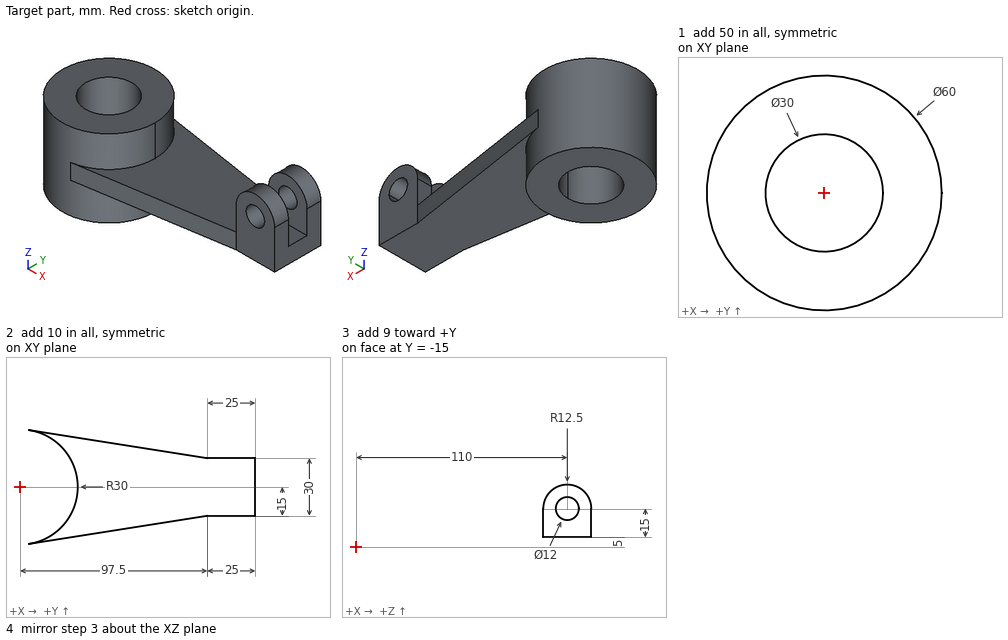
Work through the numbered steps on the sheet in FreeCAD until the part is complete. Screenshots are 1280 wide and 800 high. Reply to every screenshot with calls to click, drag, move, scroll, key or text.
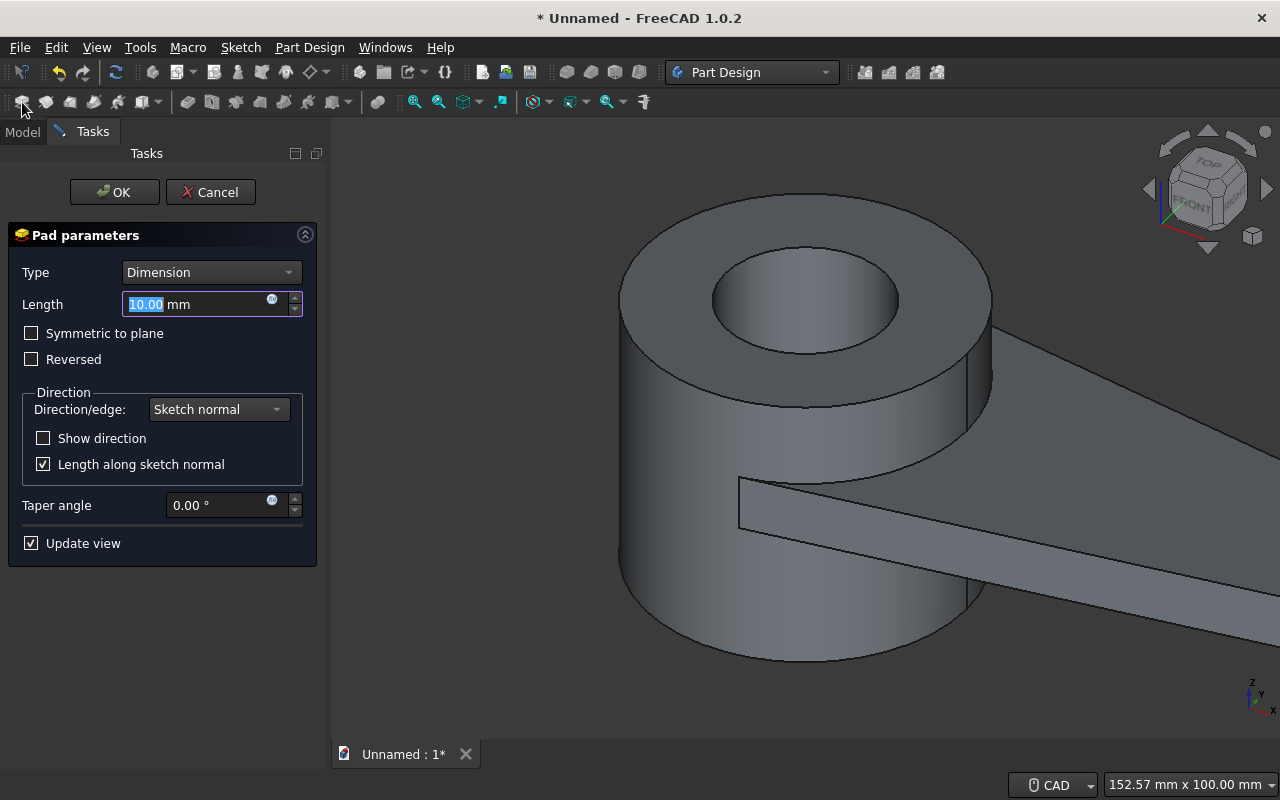
text(10)
key(Tab)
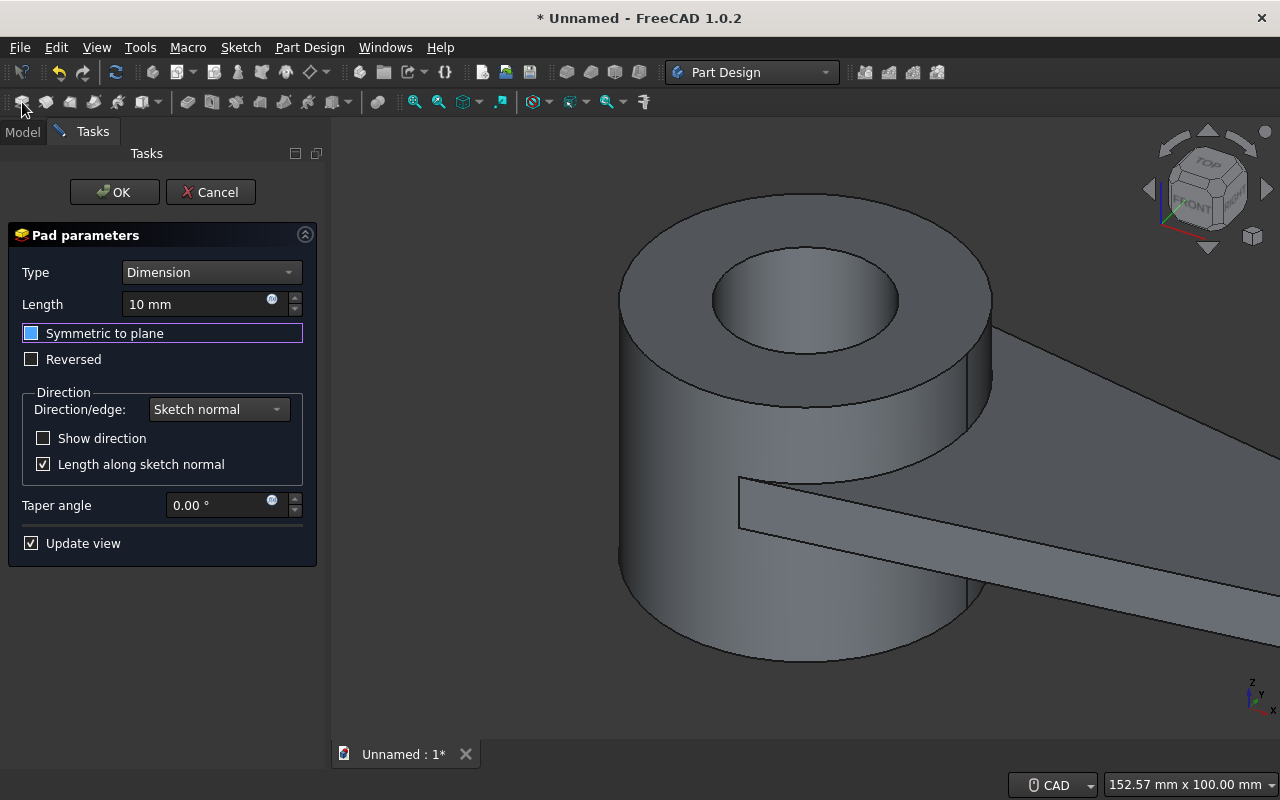
click(30, 333)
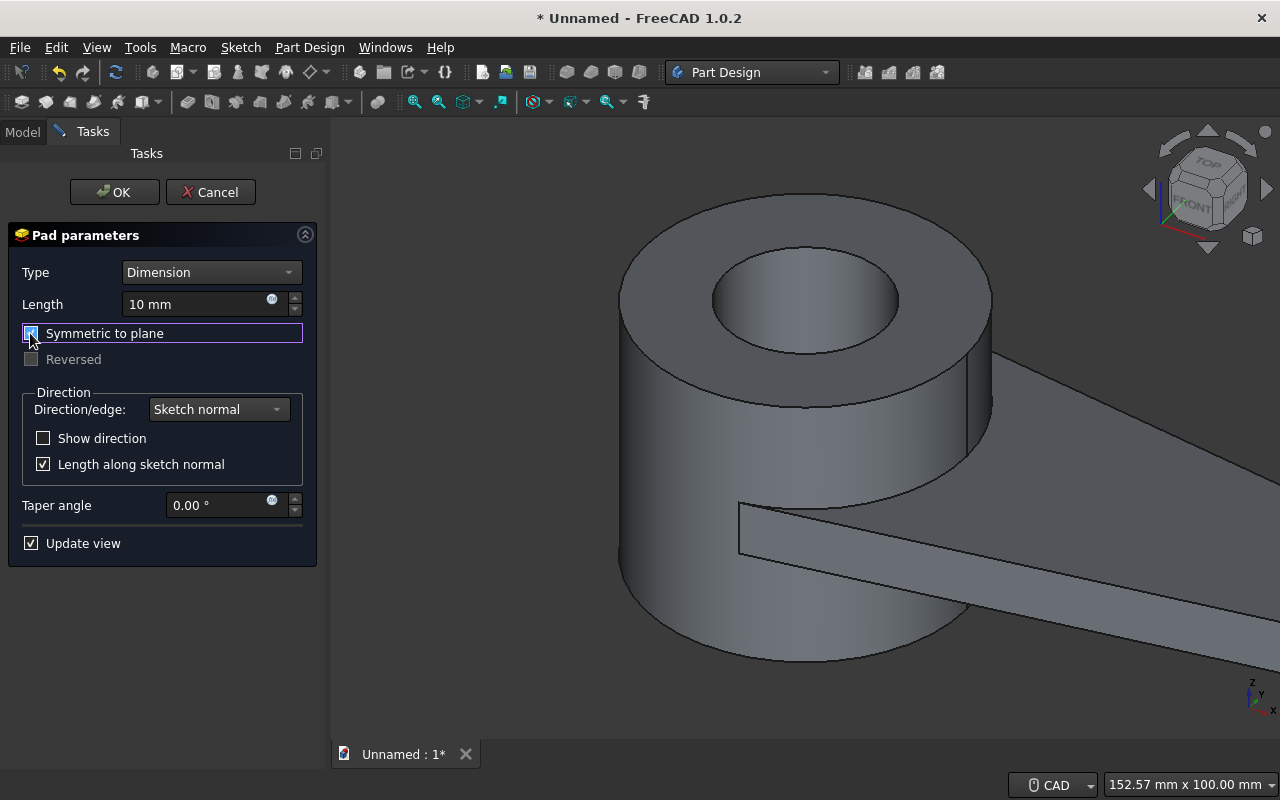
click(115, 192)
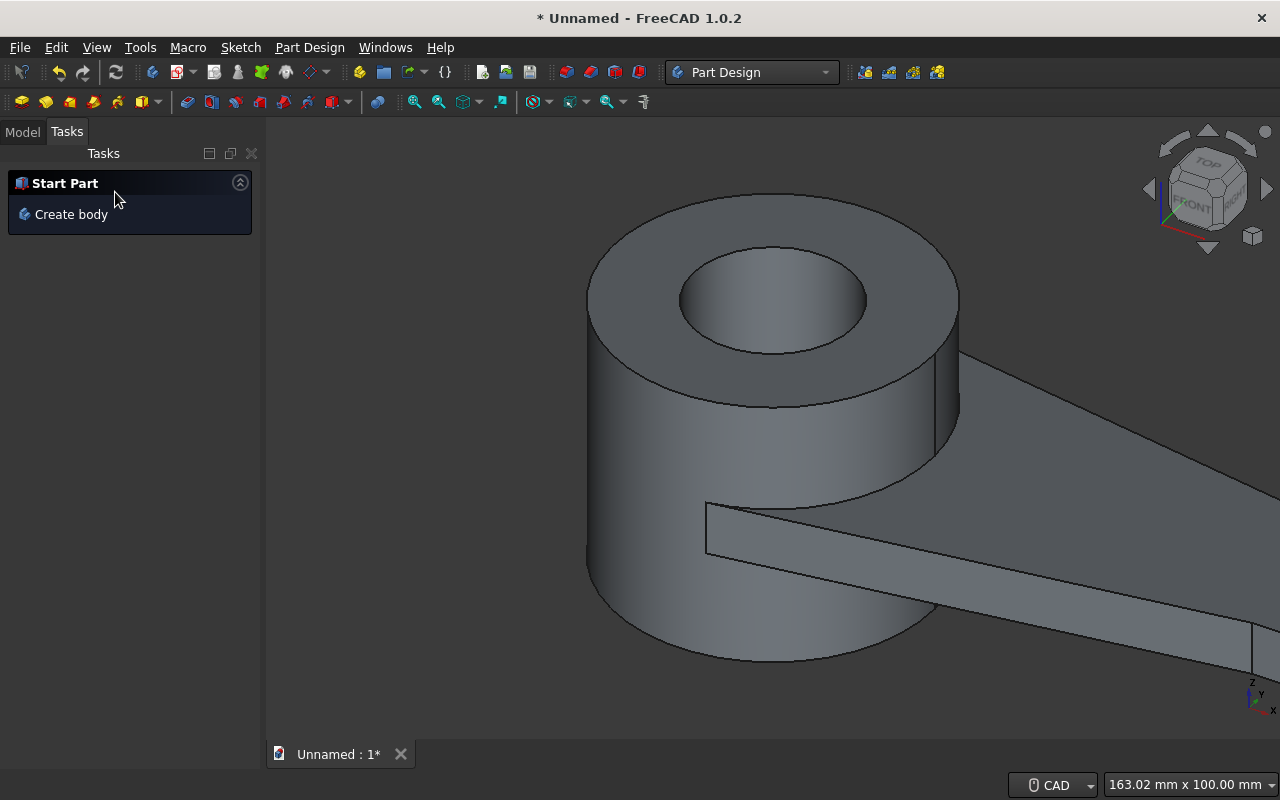
click(416, 102)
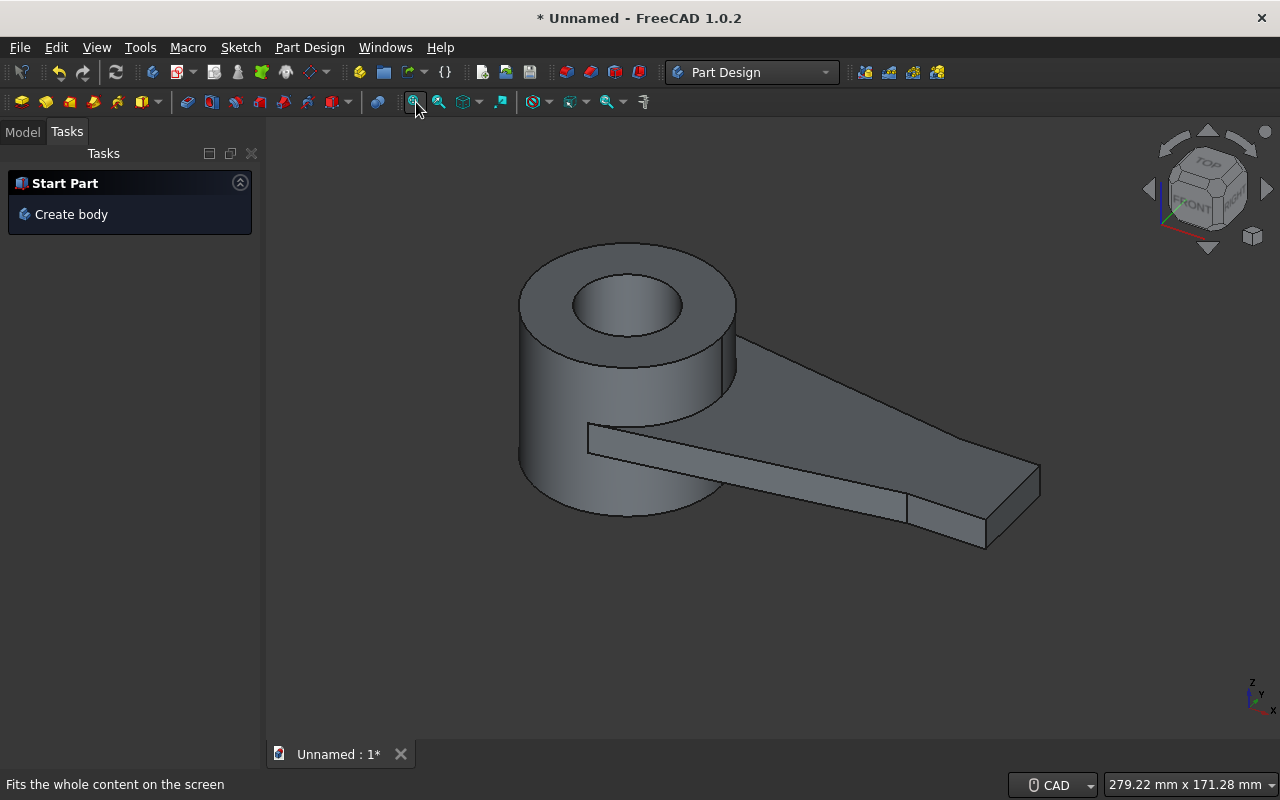
click(969, 528)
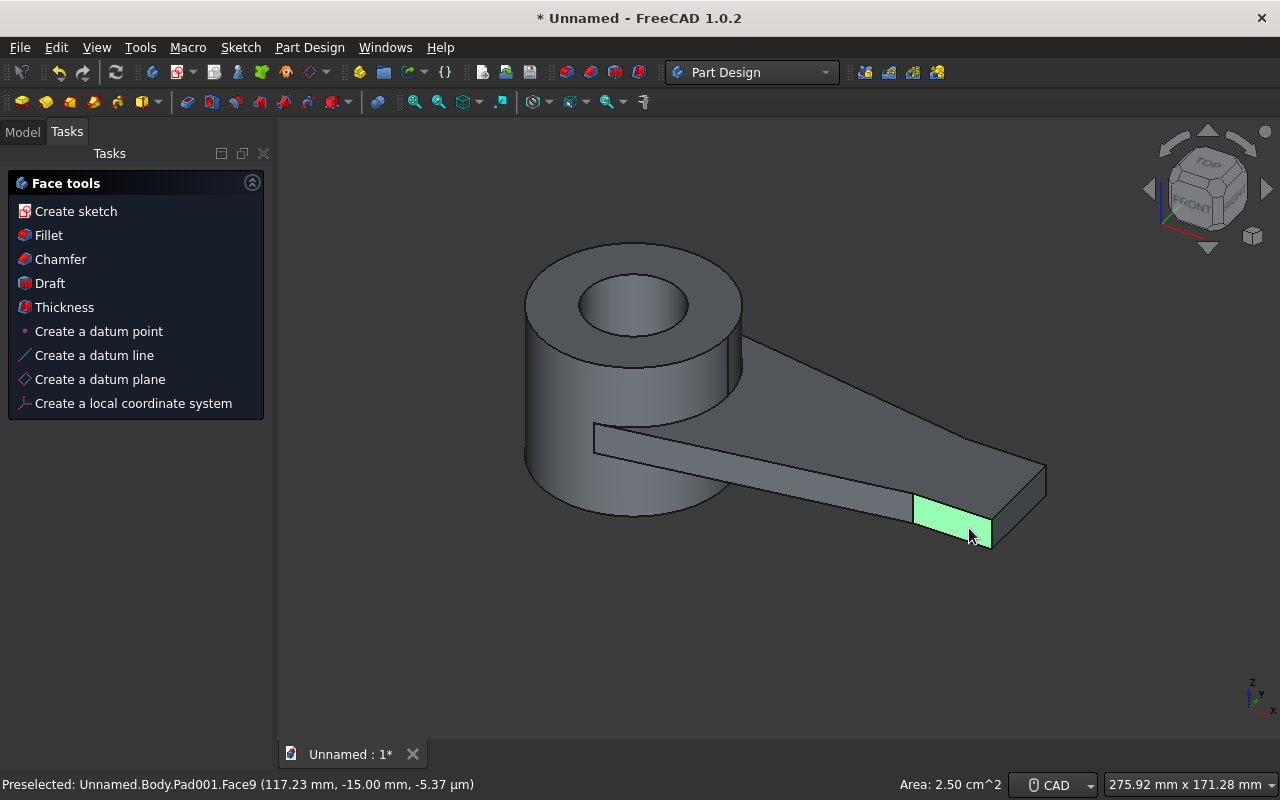
click(178, 72)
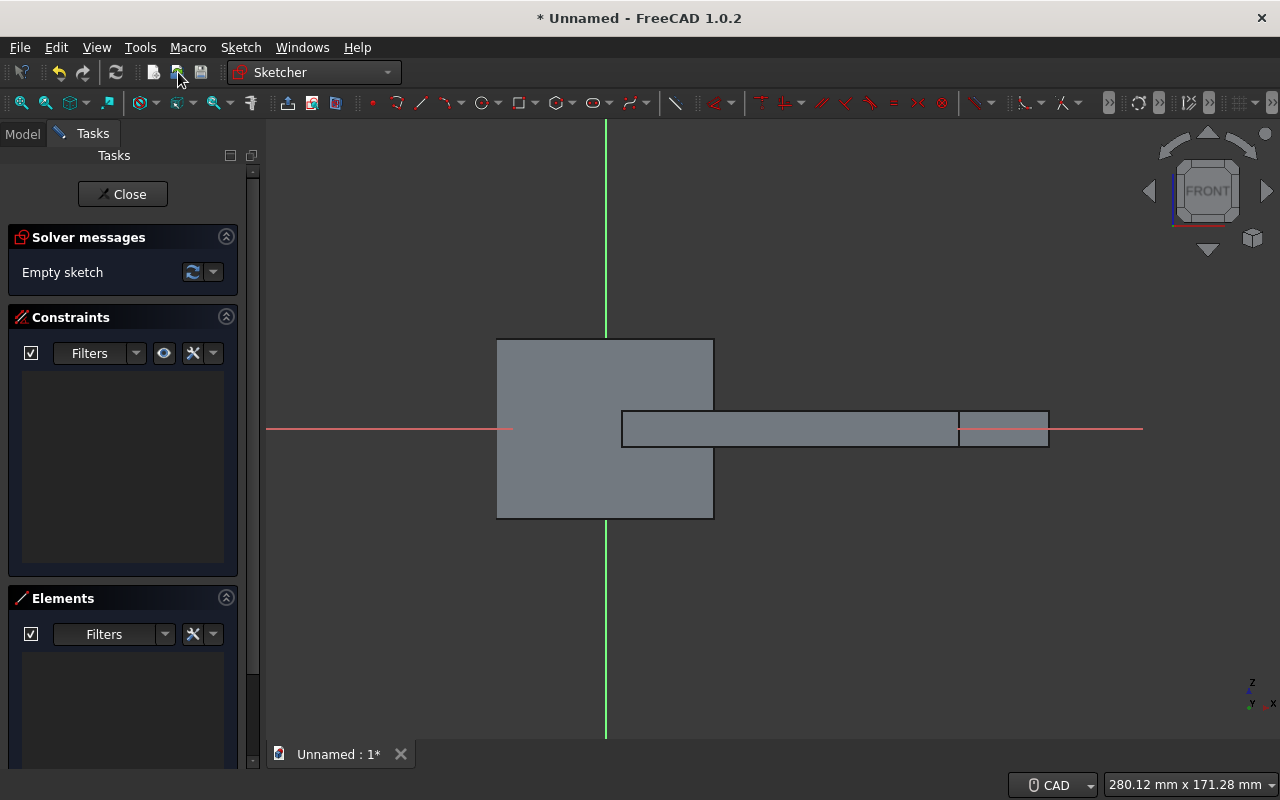
scroll(1102, 339, up, 7)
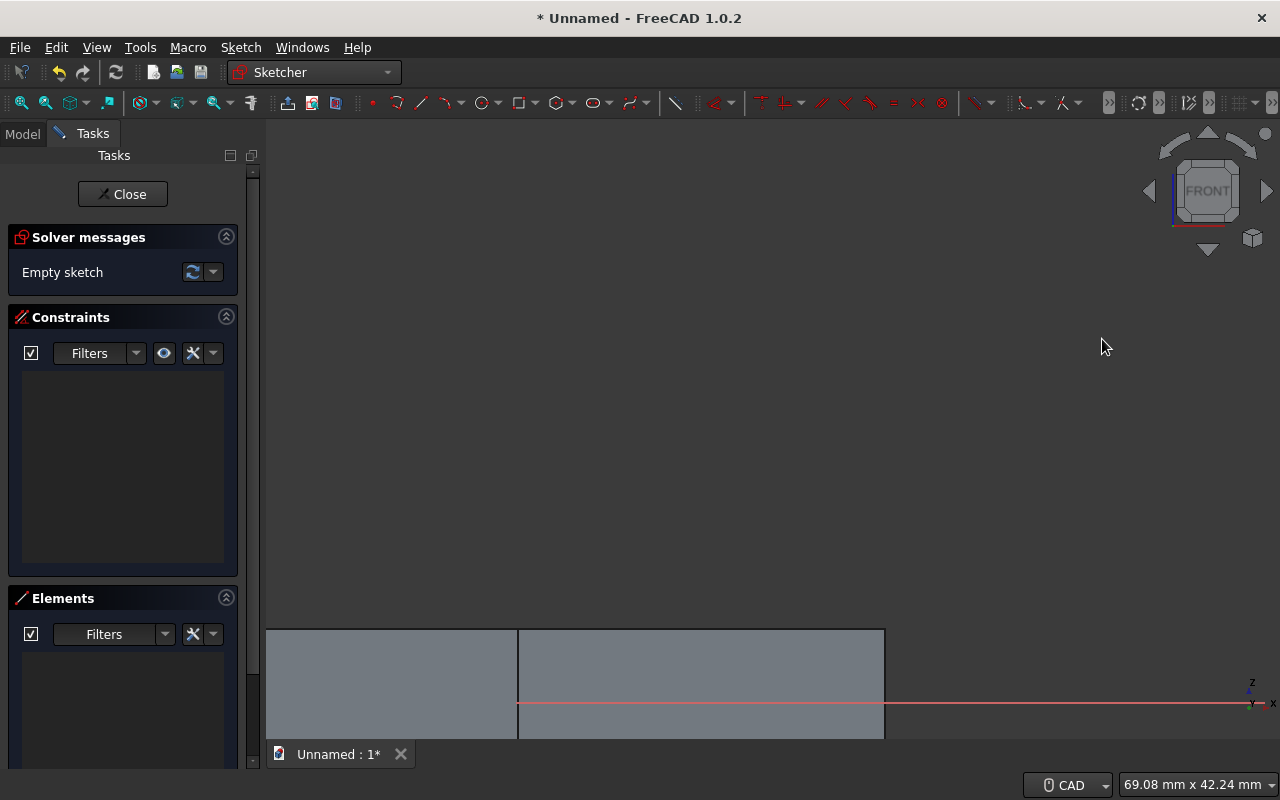
click(398, 104)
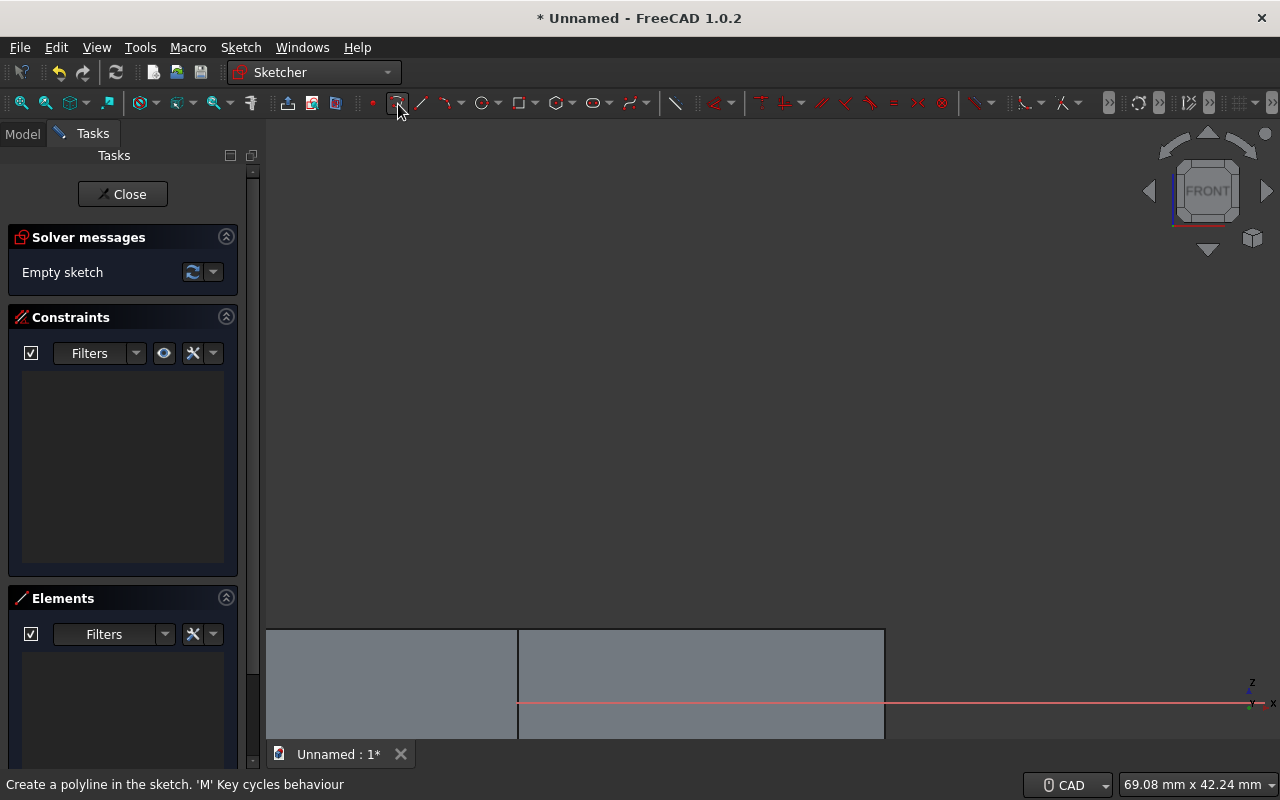
click(518, 409)
click(518, 629)
click(885, 629)
click(885, 409)
right_click(885, 409)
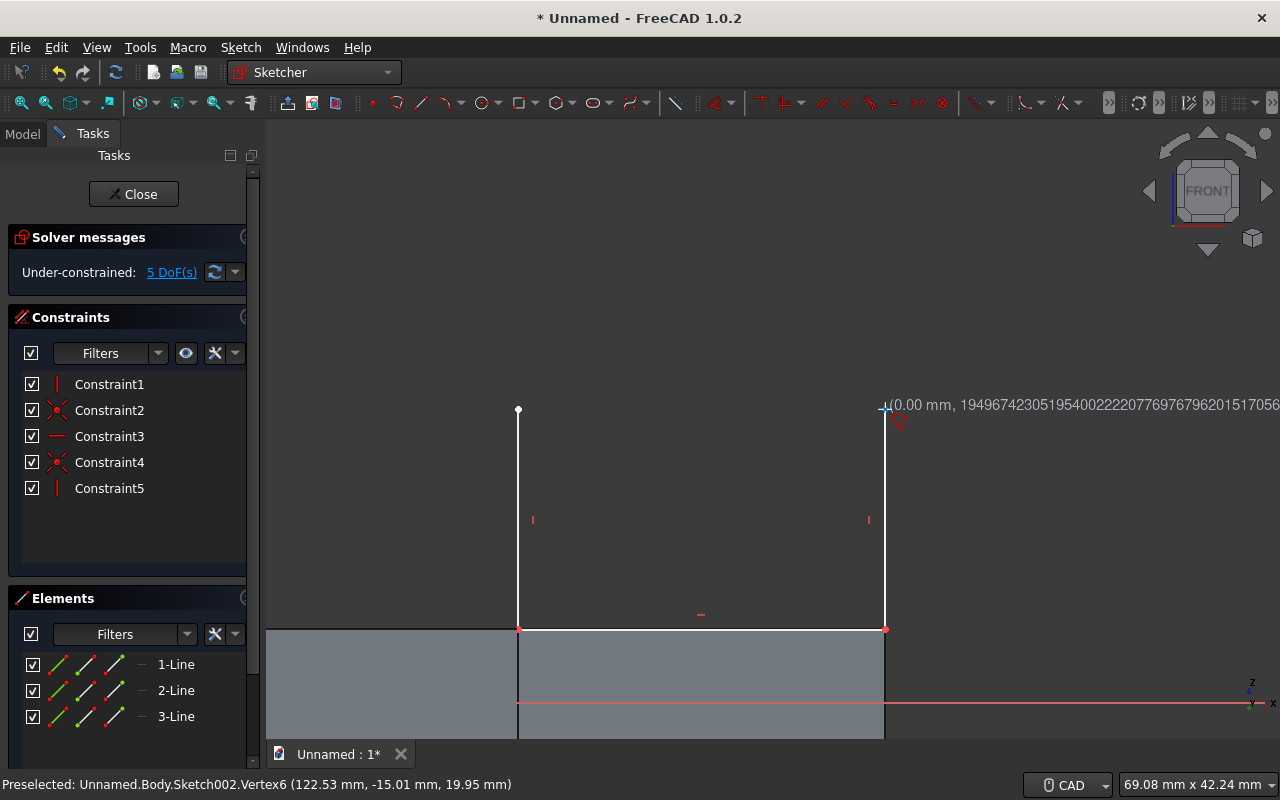
click(446, 104)